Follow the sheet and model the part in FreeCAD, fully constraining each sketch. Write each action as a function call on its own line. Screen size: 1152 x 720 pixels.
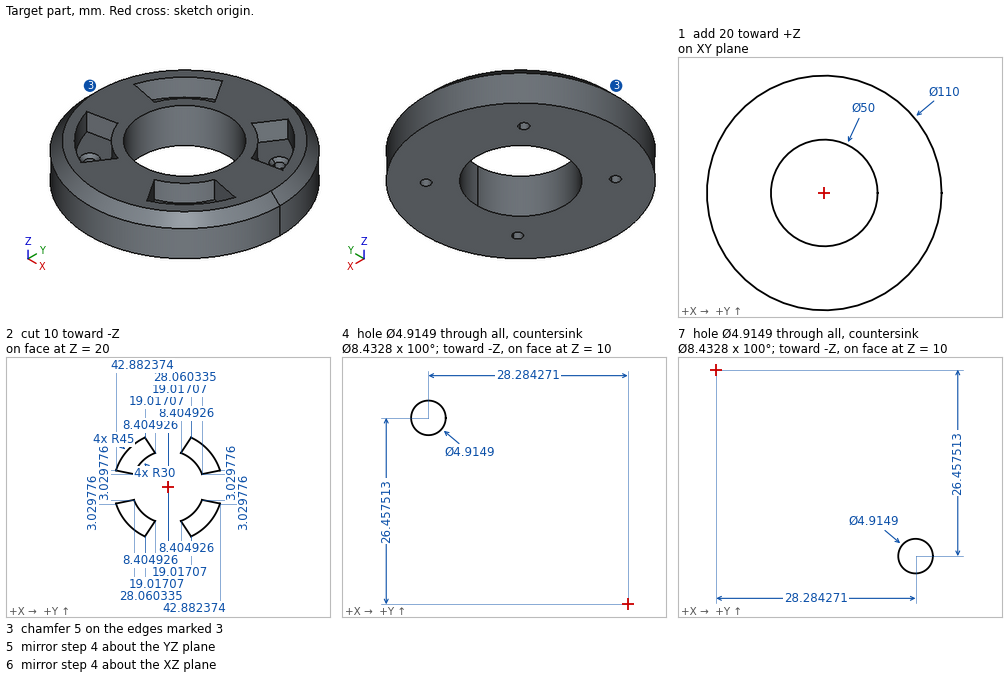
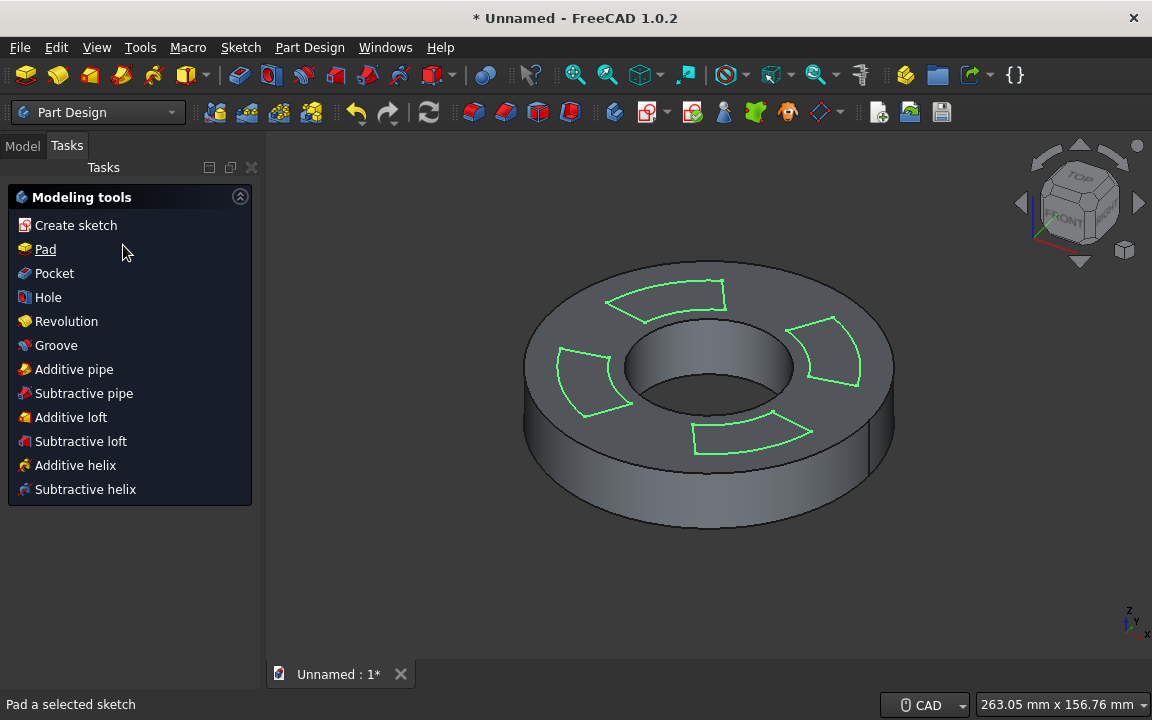
click(240, 76)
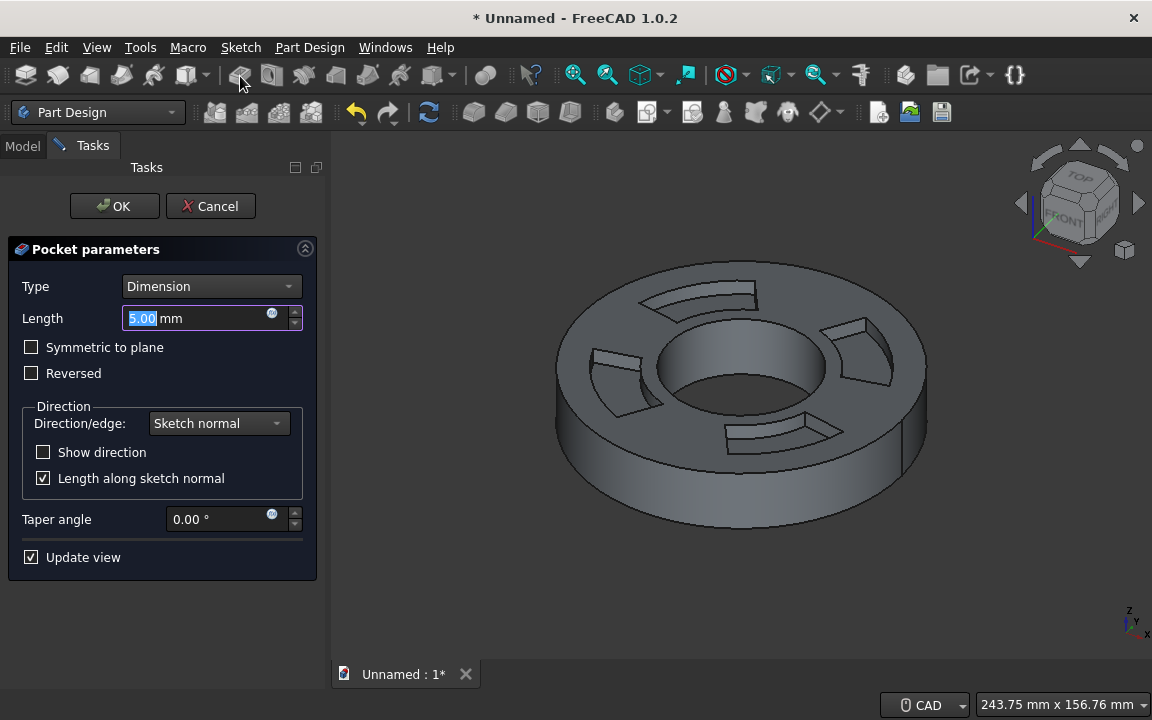
text(10)
key(Tab)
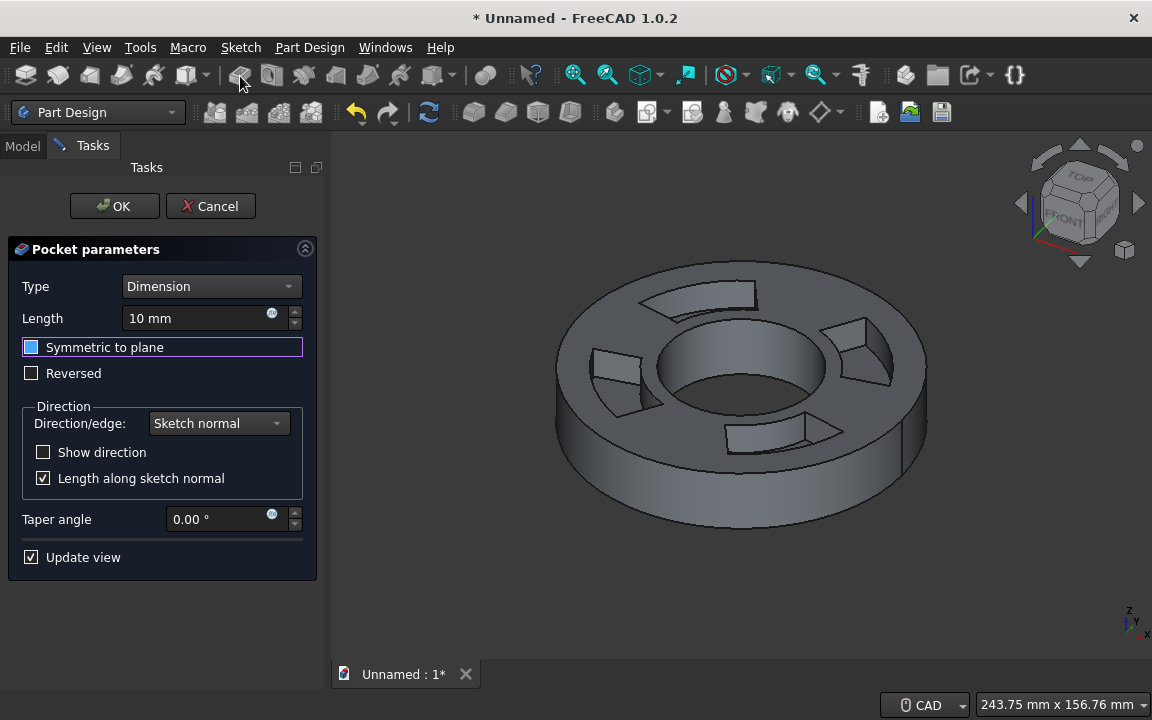
click(115, 206)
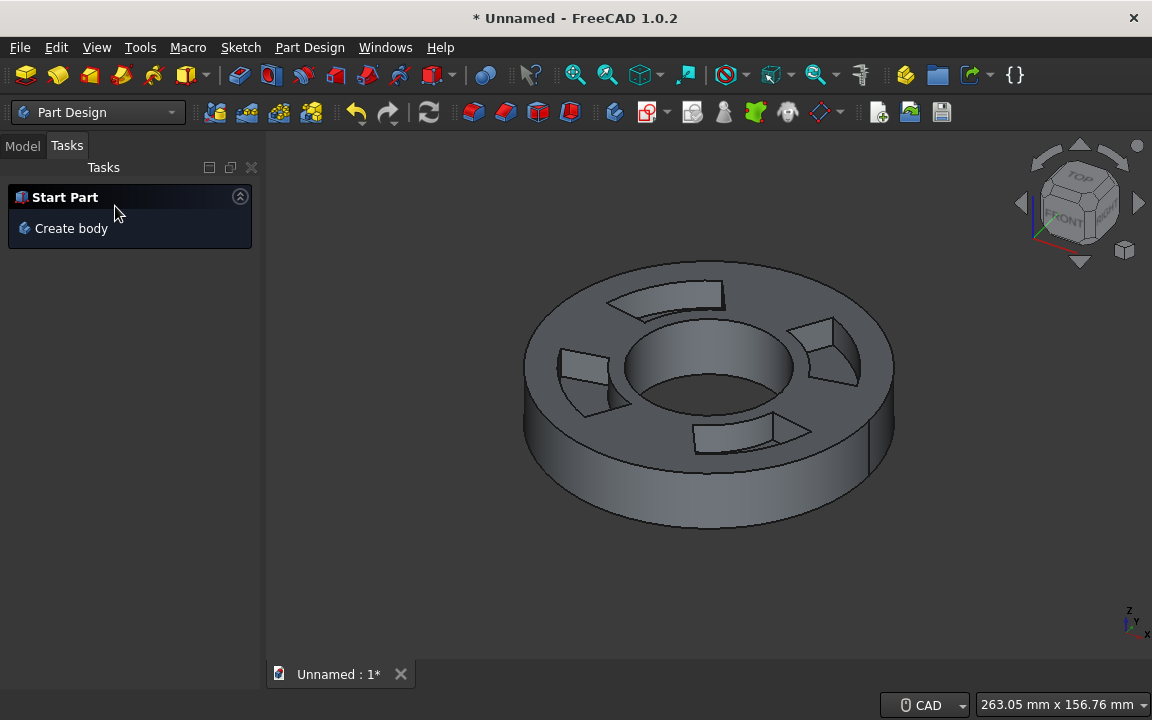
click(525, 377)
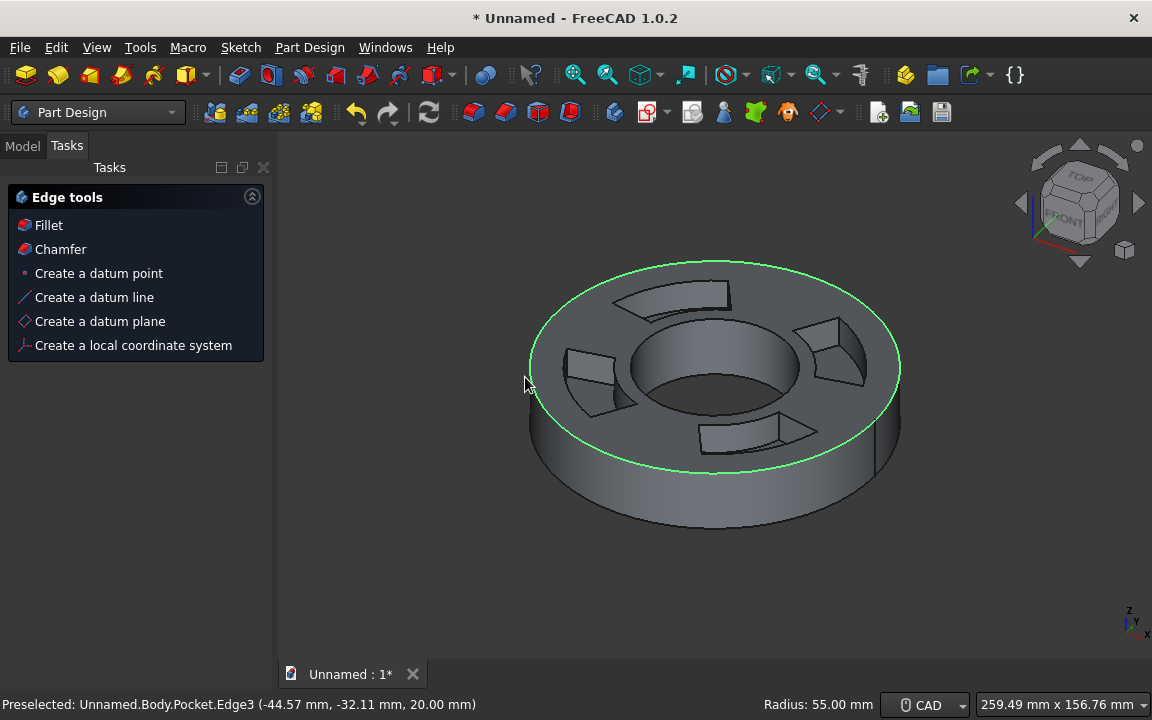
click(506, 112)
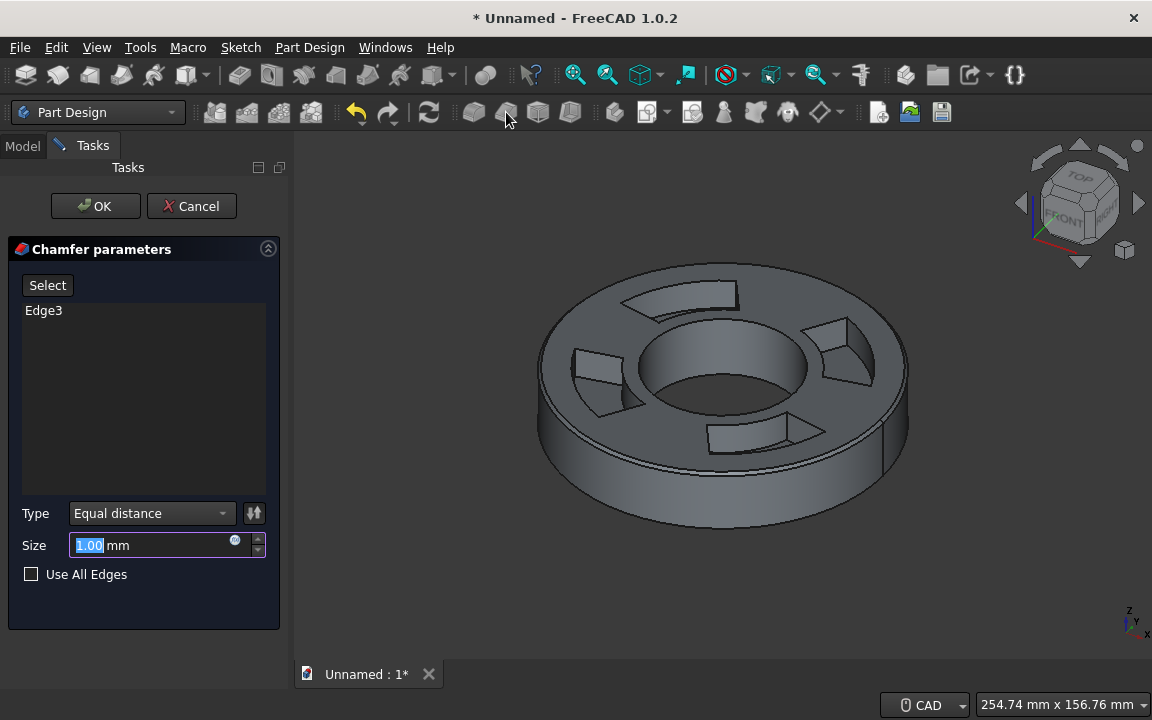
text(5)
key(Tab)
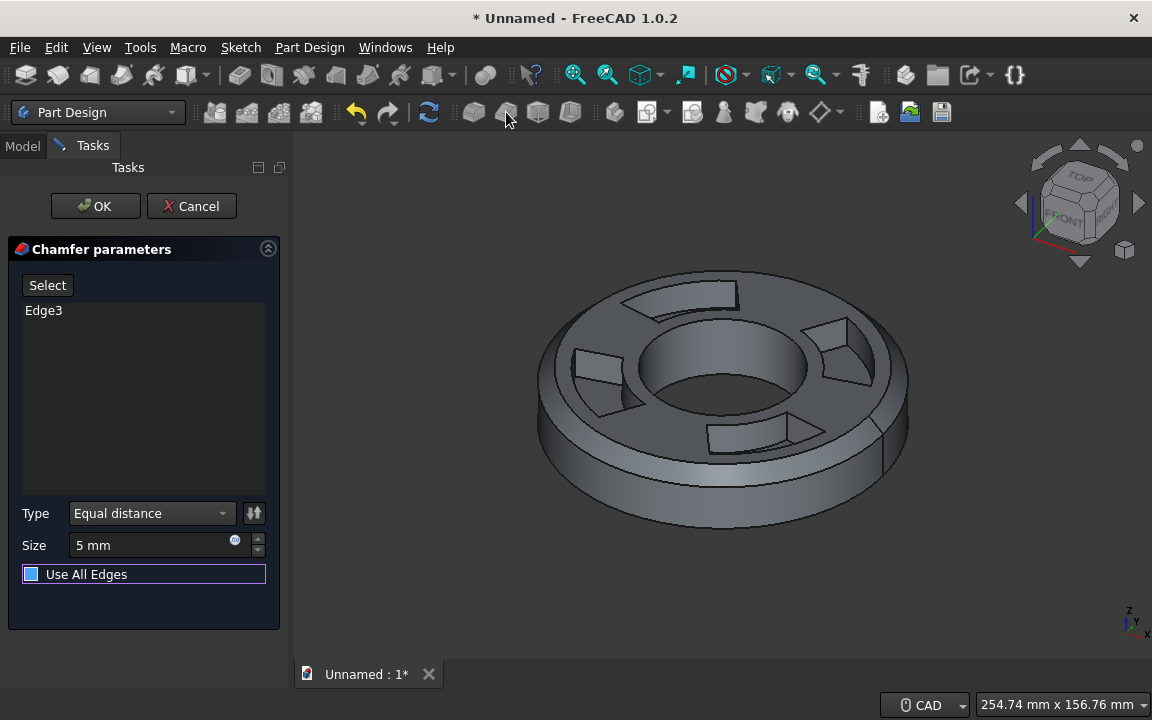
click(96, 206)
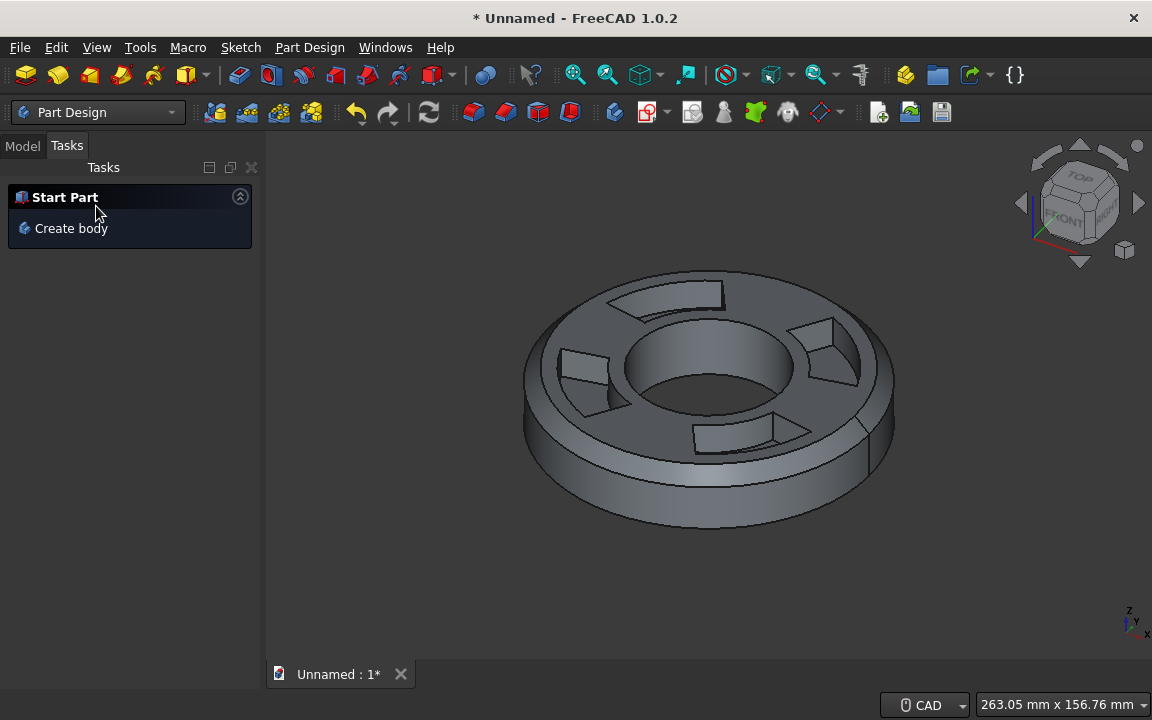
click(824, 365)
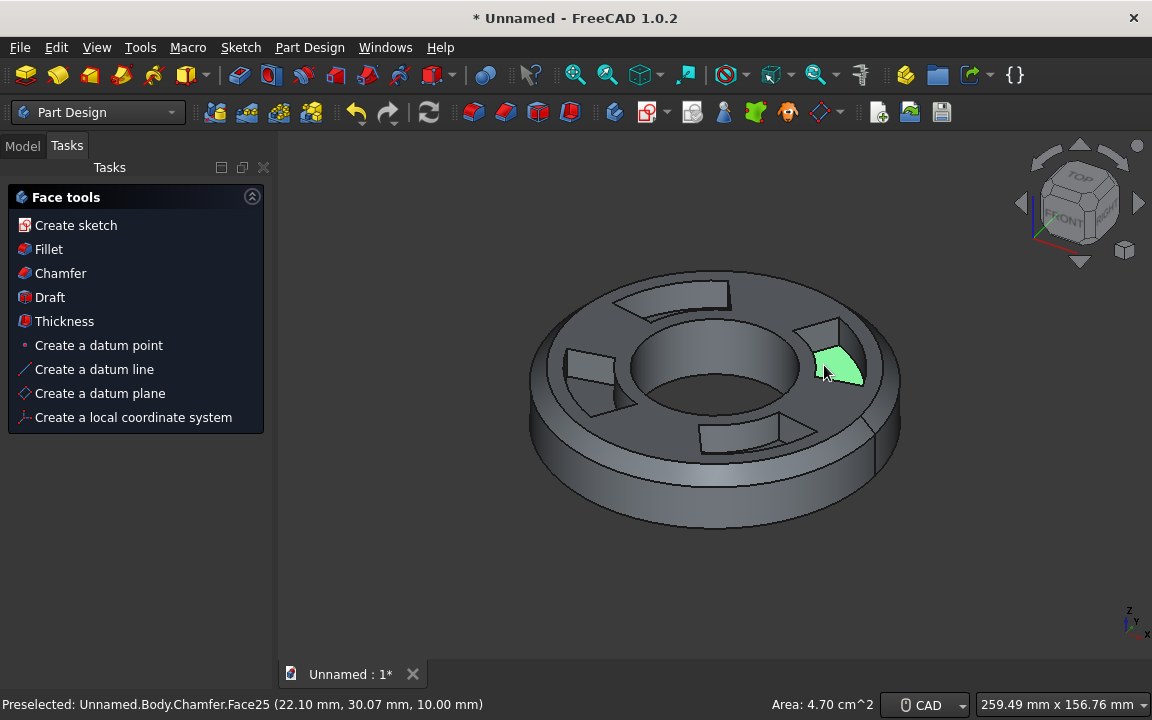
click(648, 112)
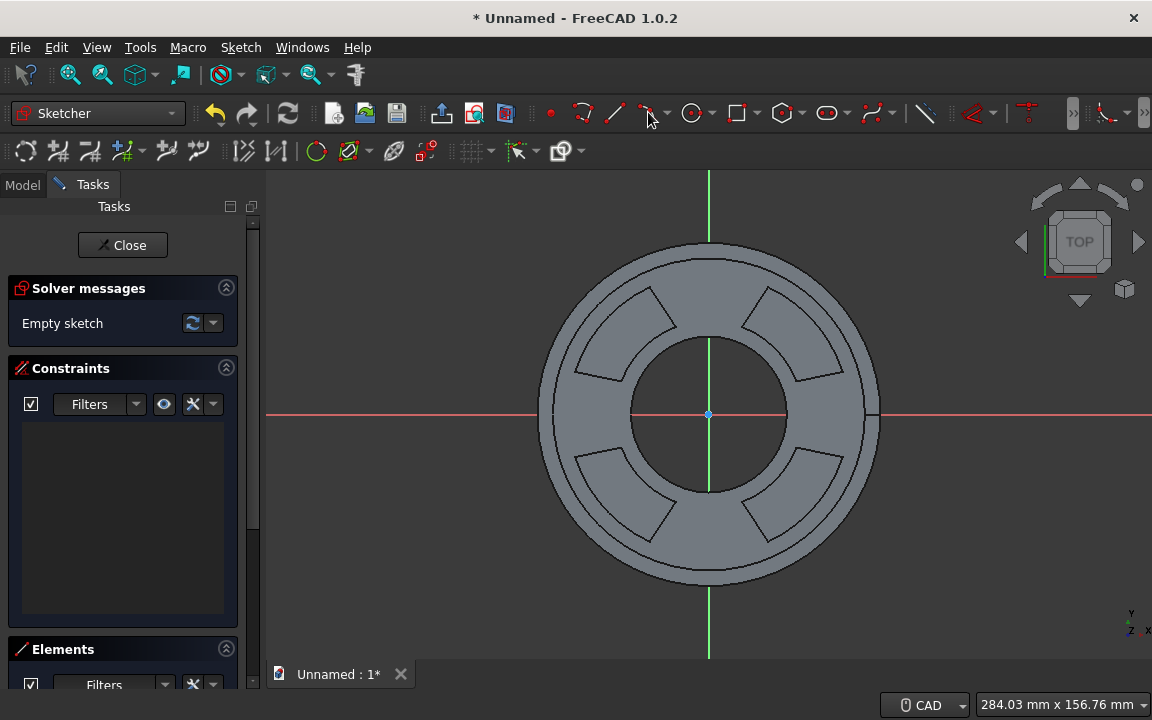
click(506, 114)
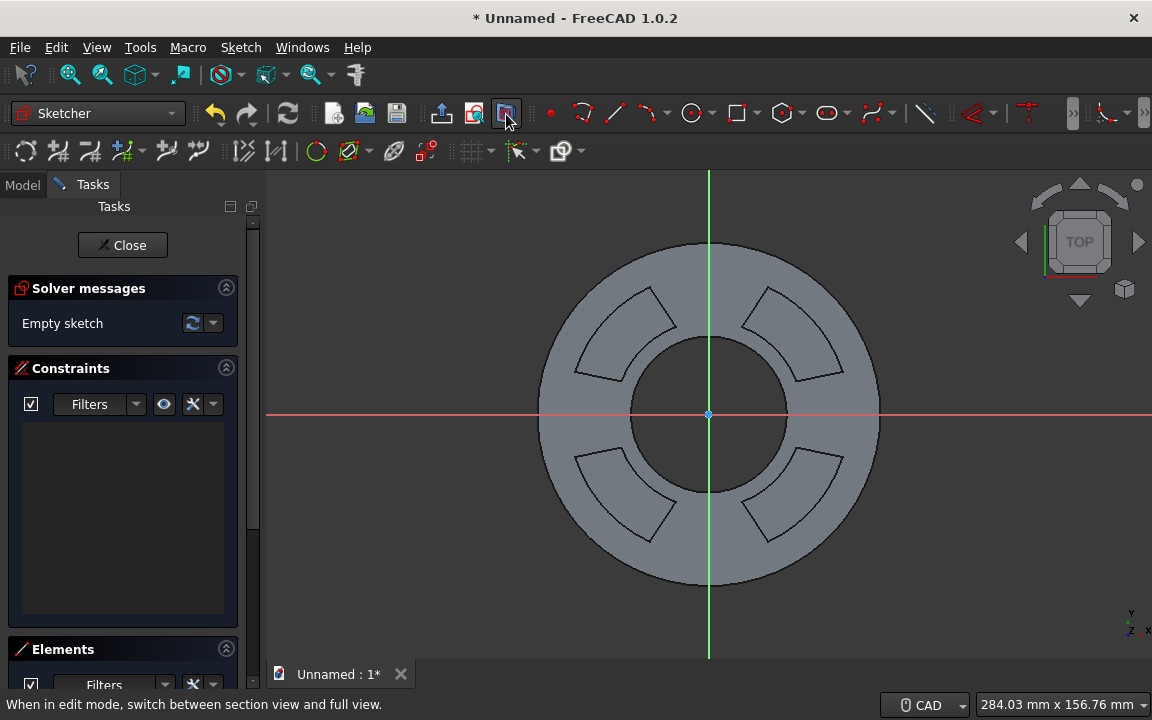
scroll(620, 328, up, 15)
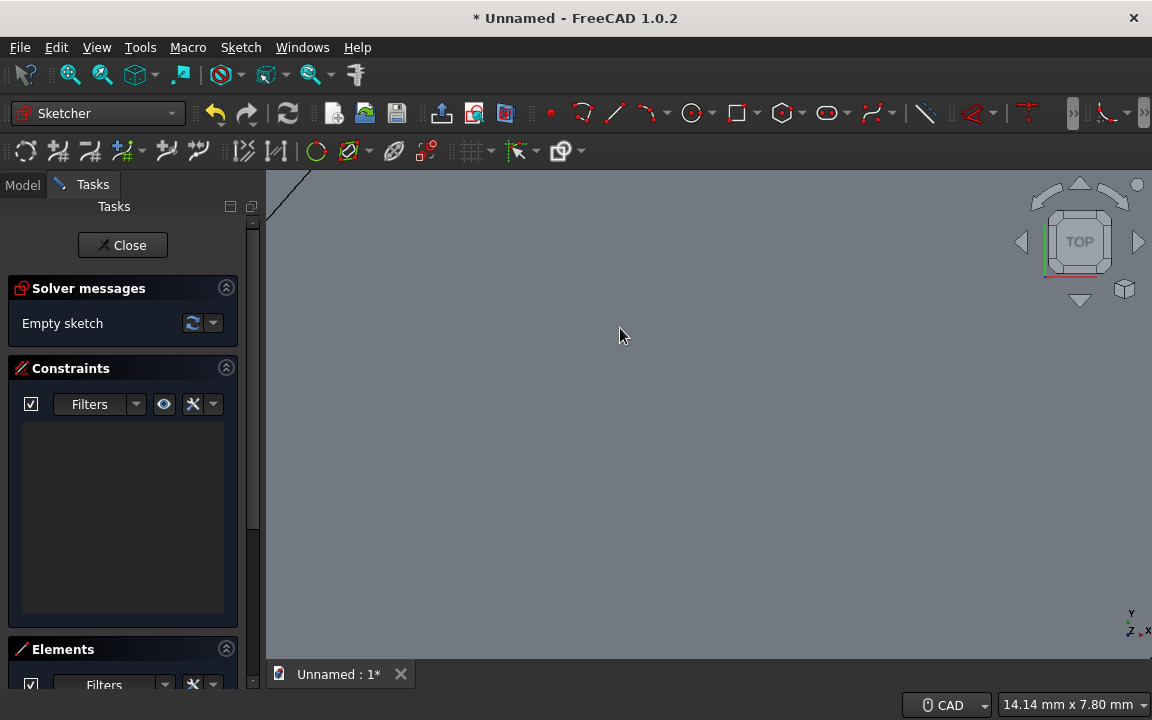
click(692, 114)